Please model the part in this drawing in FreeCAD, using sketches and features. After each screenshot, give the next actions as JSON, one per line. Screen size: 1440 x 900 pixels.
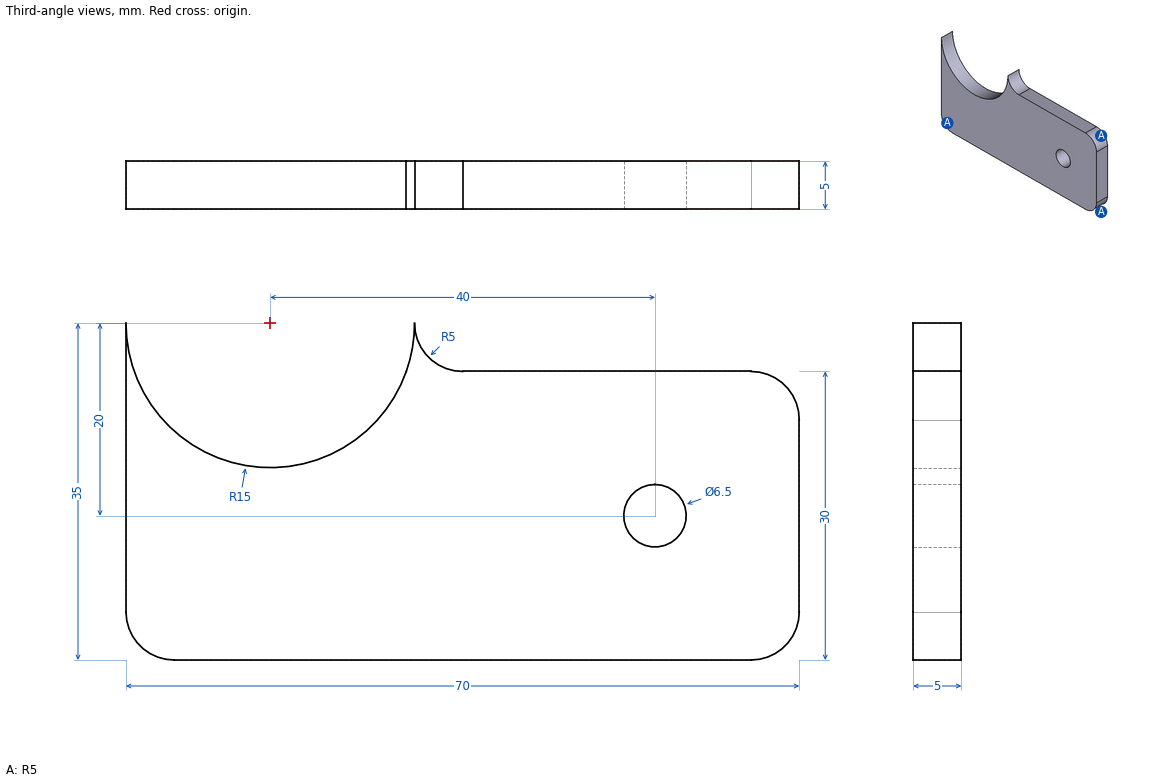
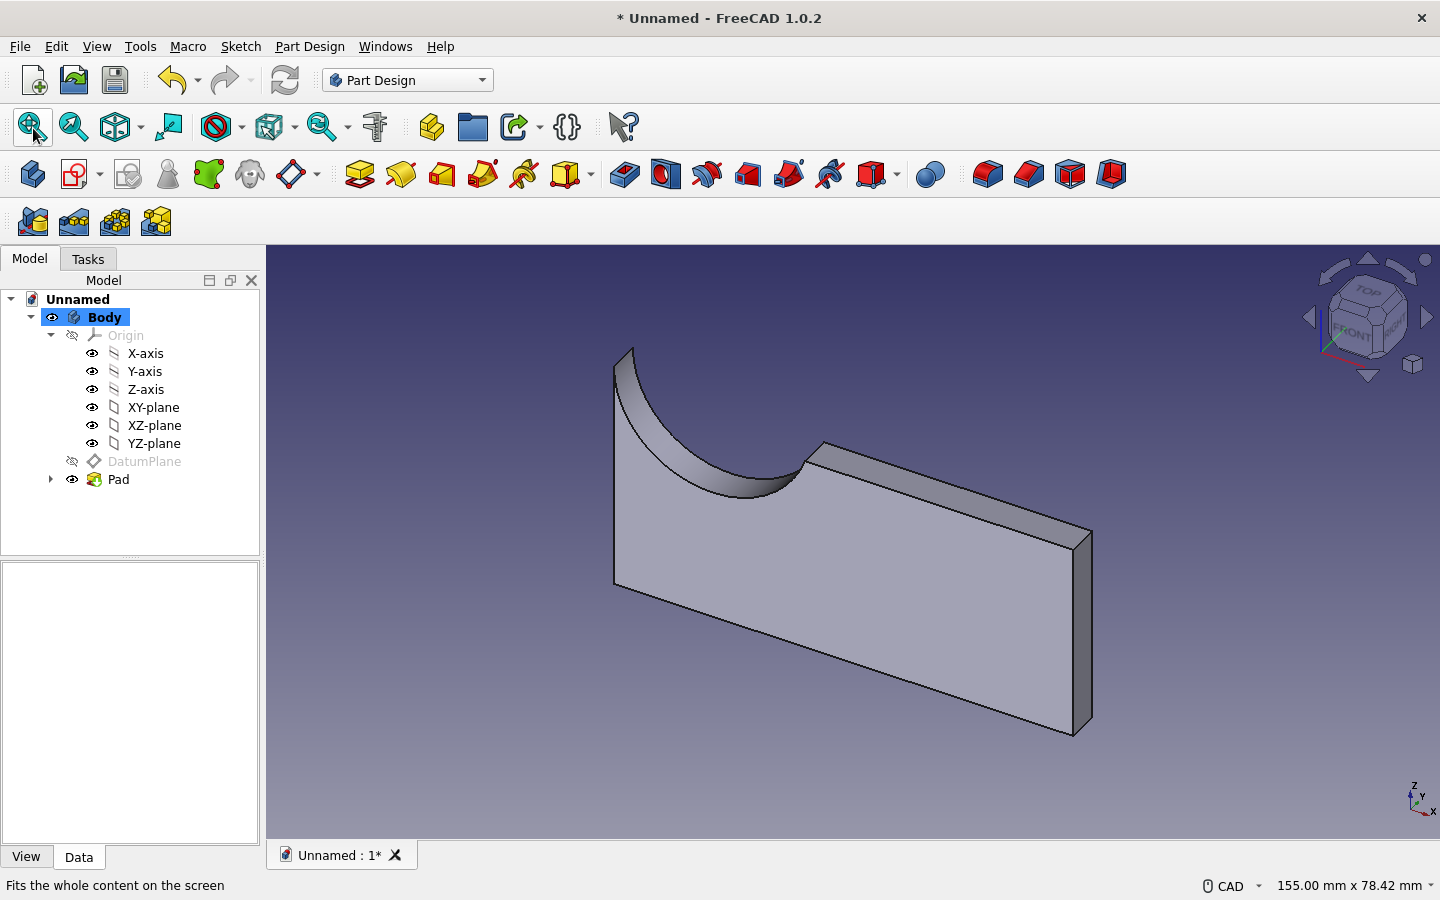
{"action": "left_click", "coordinate": [1083, 539]}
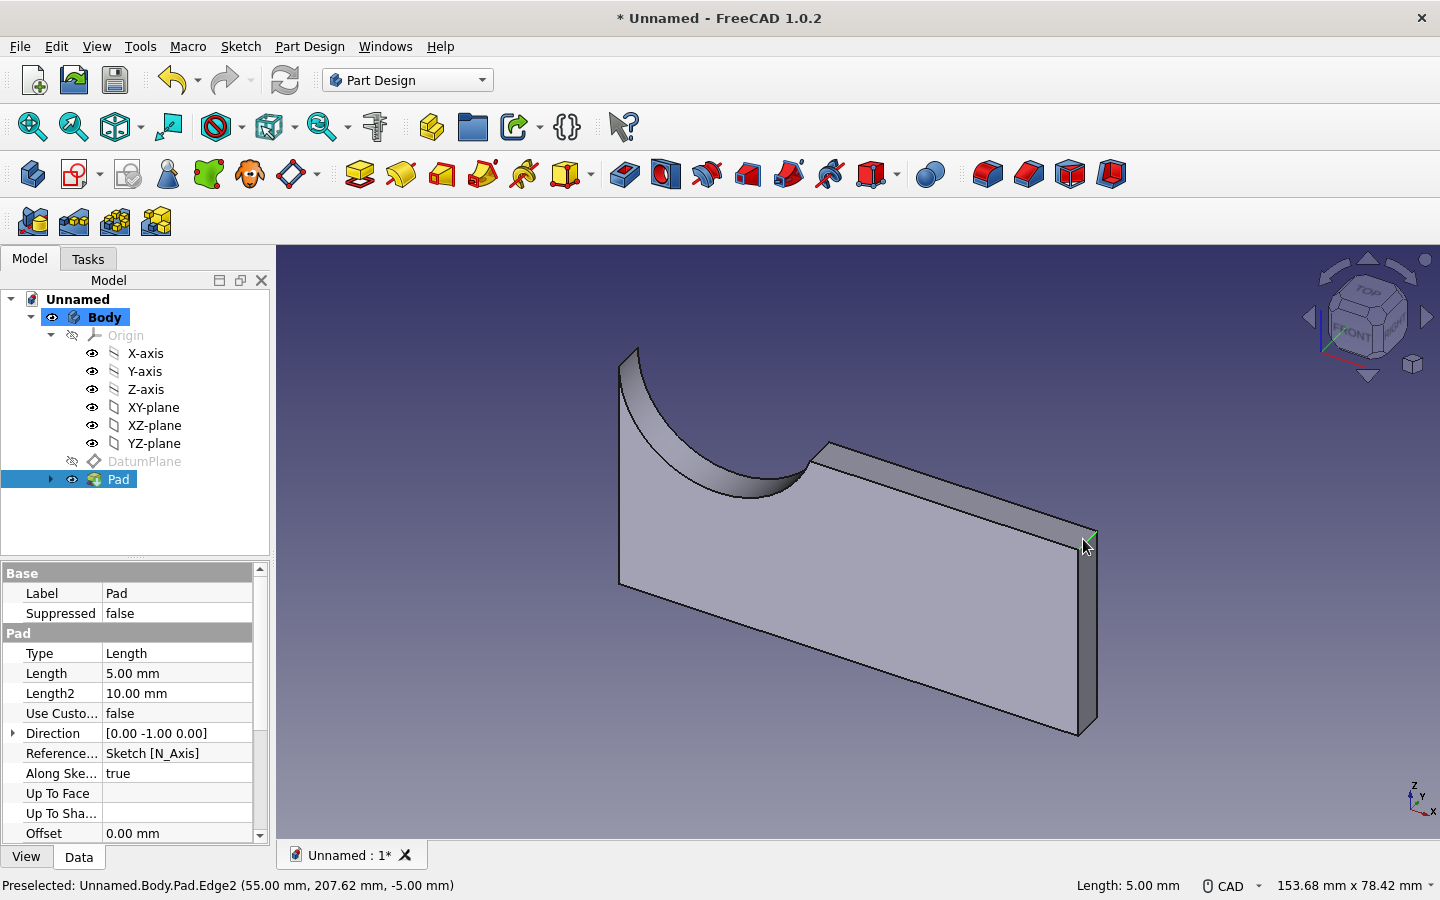
{"action": "key", "text": "0"}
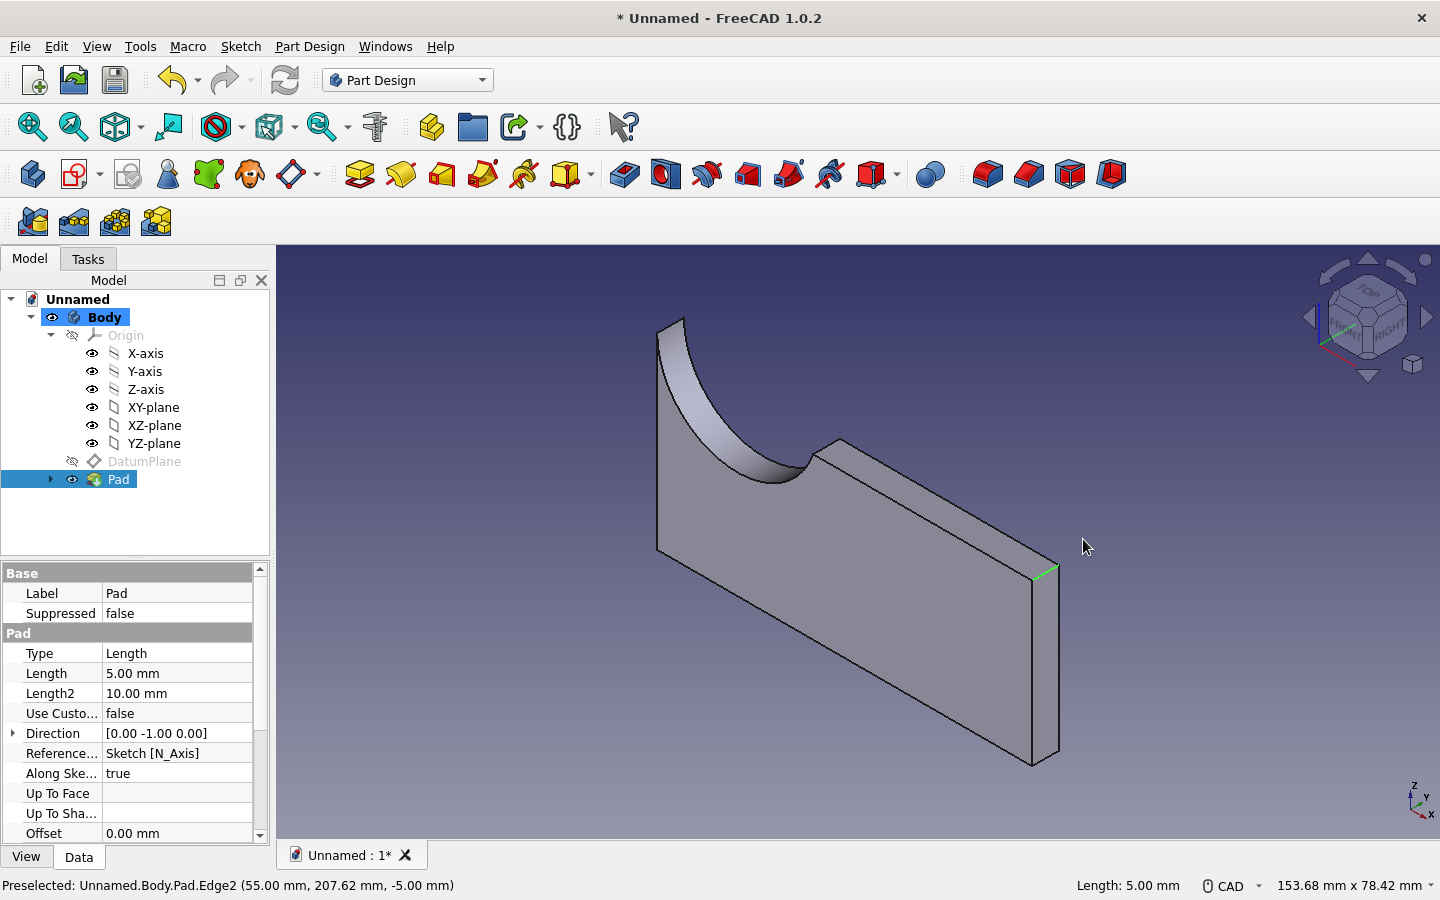
{"action": "key", "text": "2"}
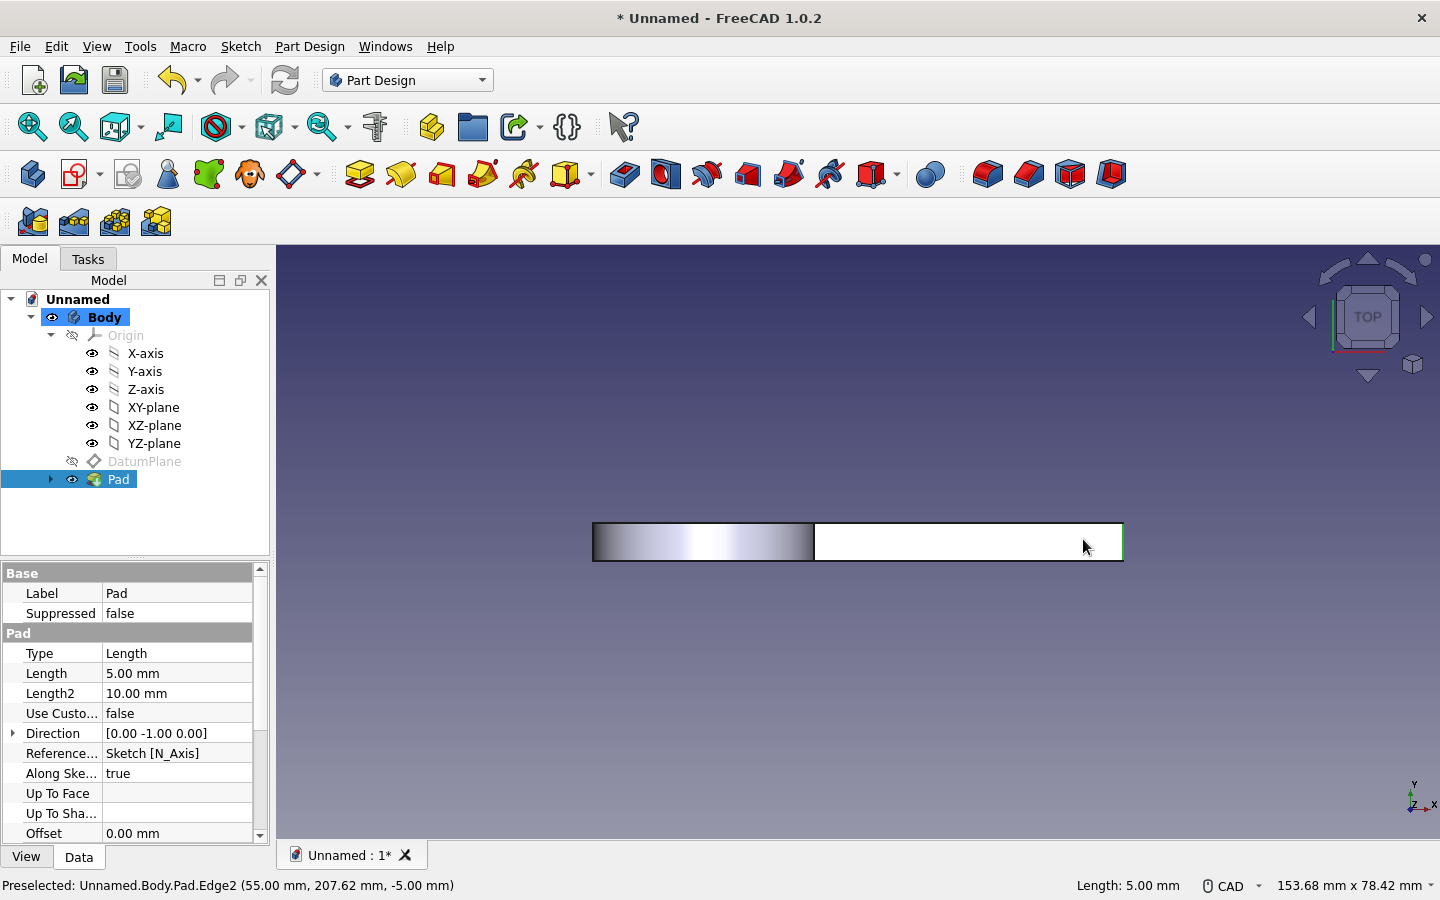
{"action": "key", "text": "1"}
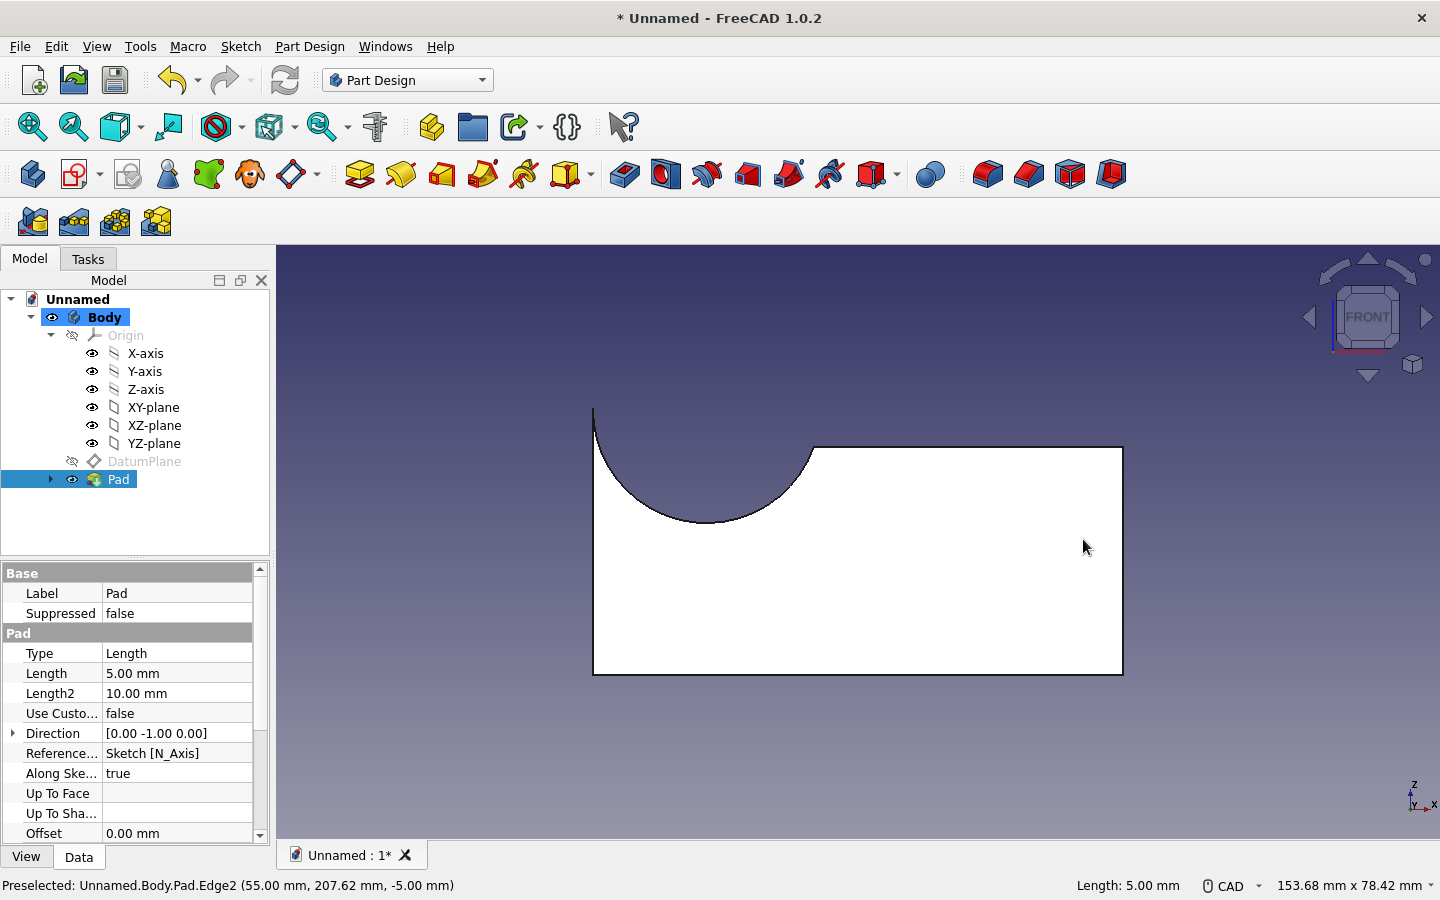
{"action": "key", "text": "3"}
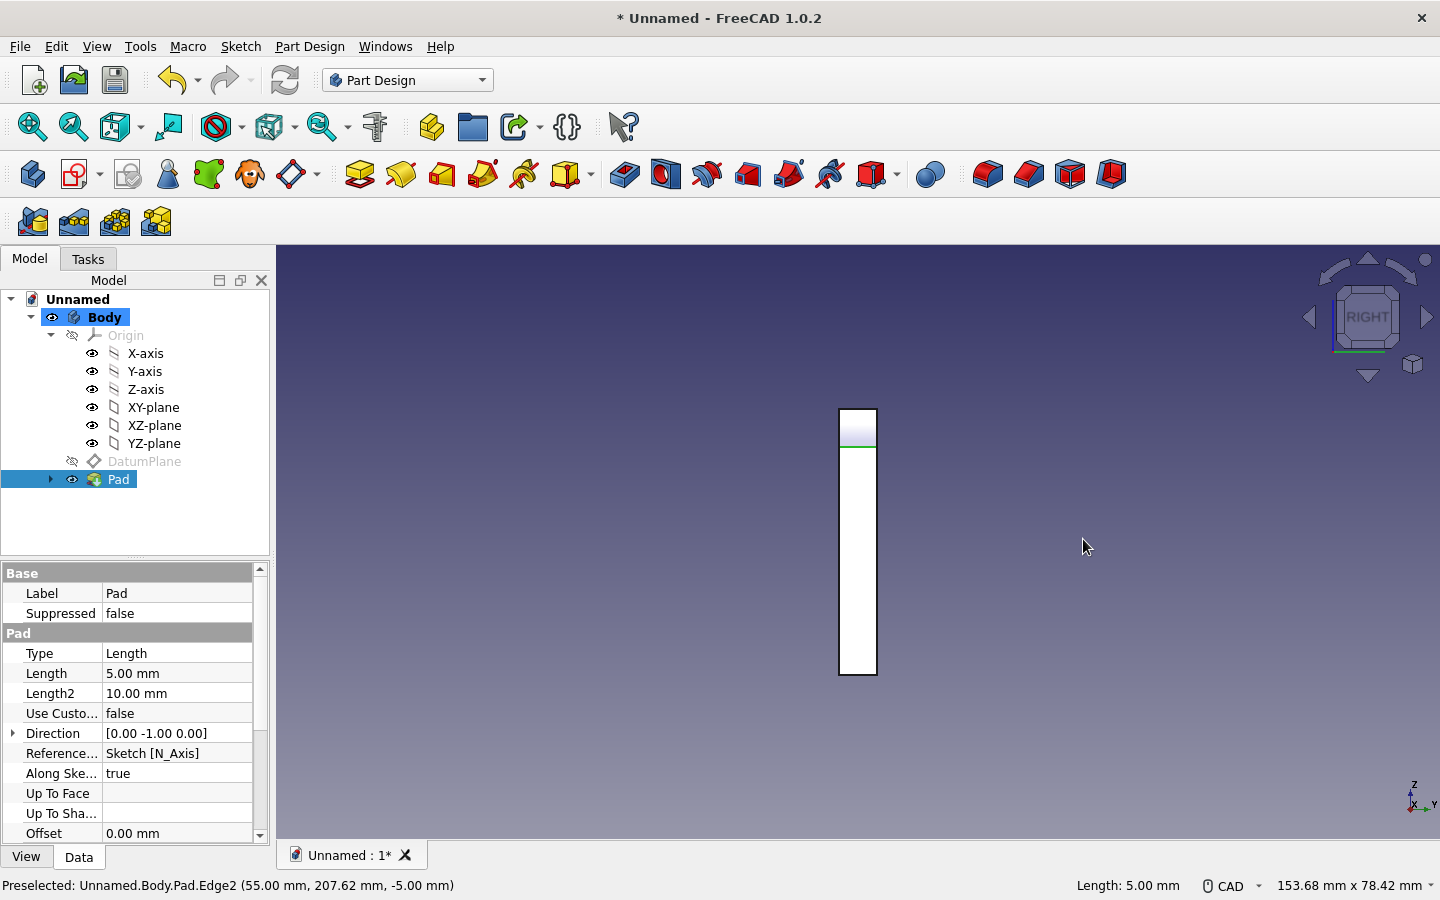
{"action": "left_click", "coordinate": [33, 128]}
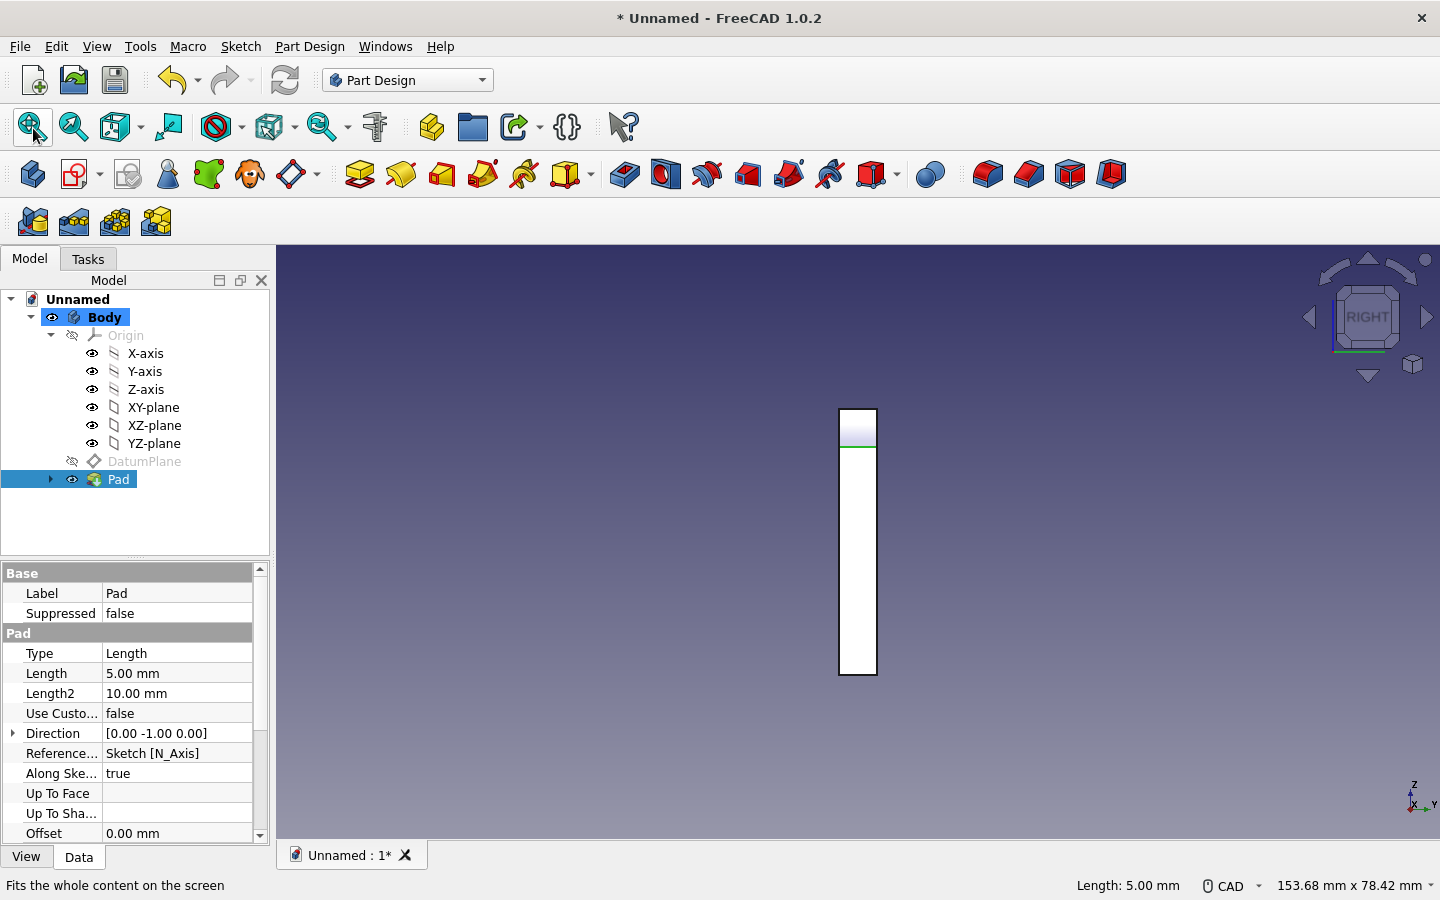
{"action": "left_click", "coordinate": [858, 674], "text": "ctrl"}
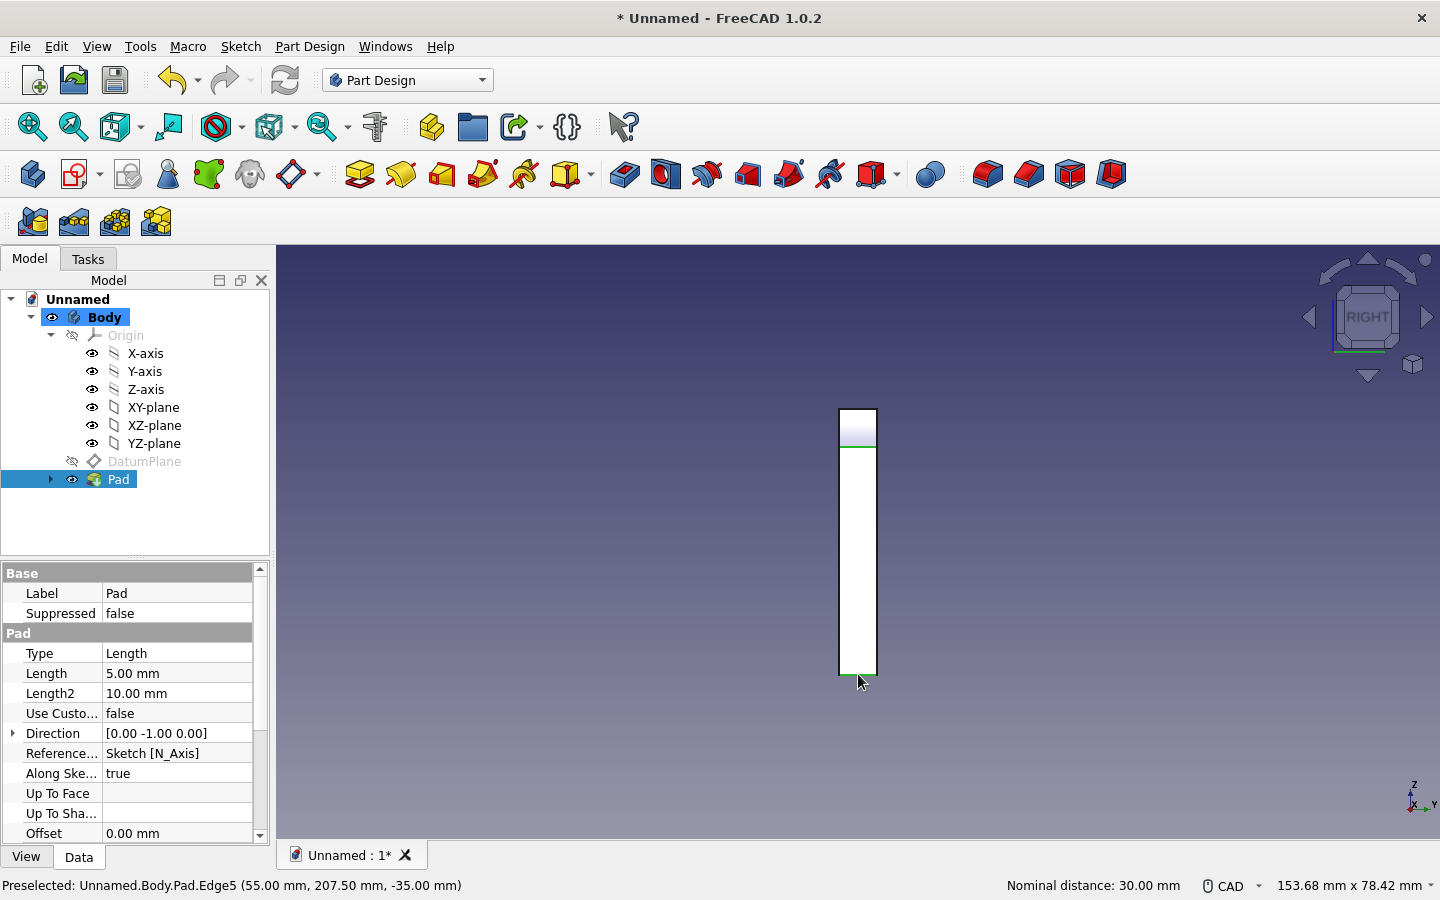
{"action": "key", "text": "5"}